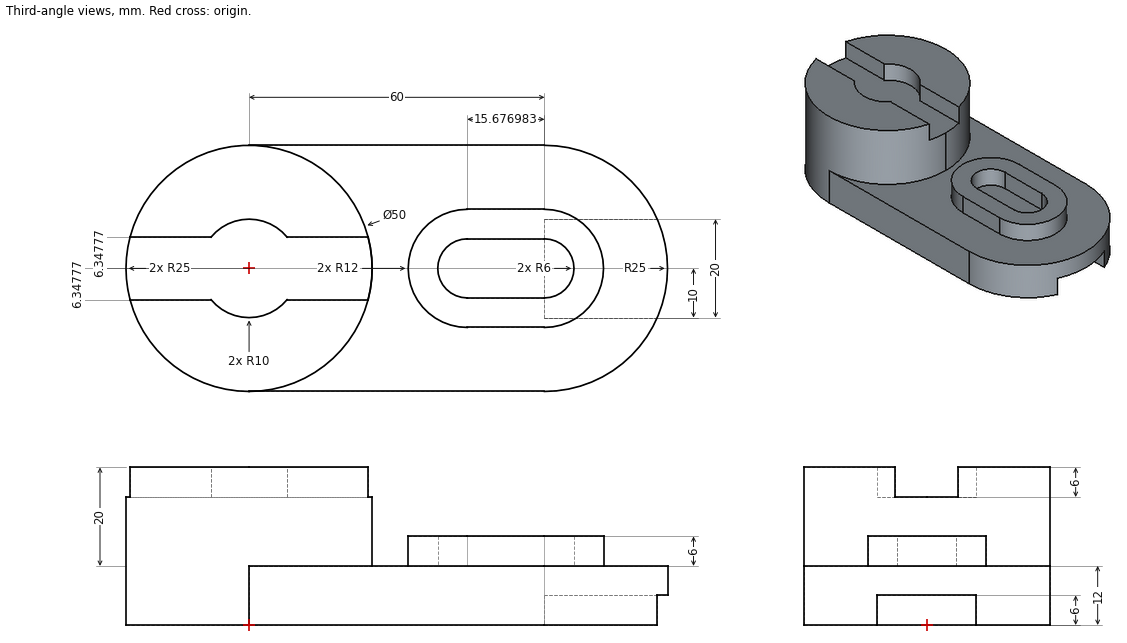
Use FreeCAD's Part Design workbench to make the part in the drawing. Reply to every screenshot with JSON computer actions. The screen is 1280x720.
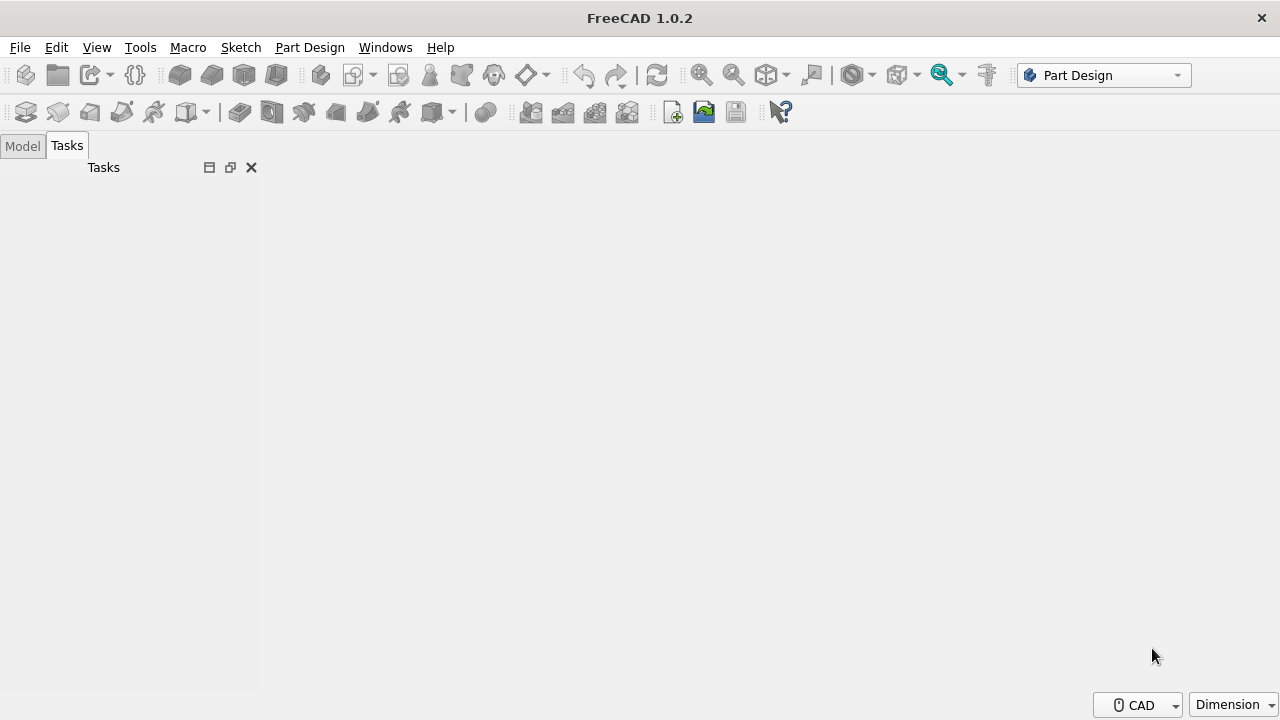
{"action": "key", "text": "ctrl+n"}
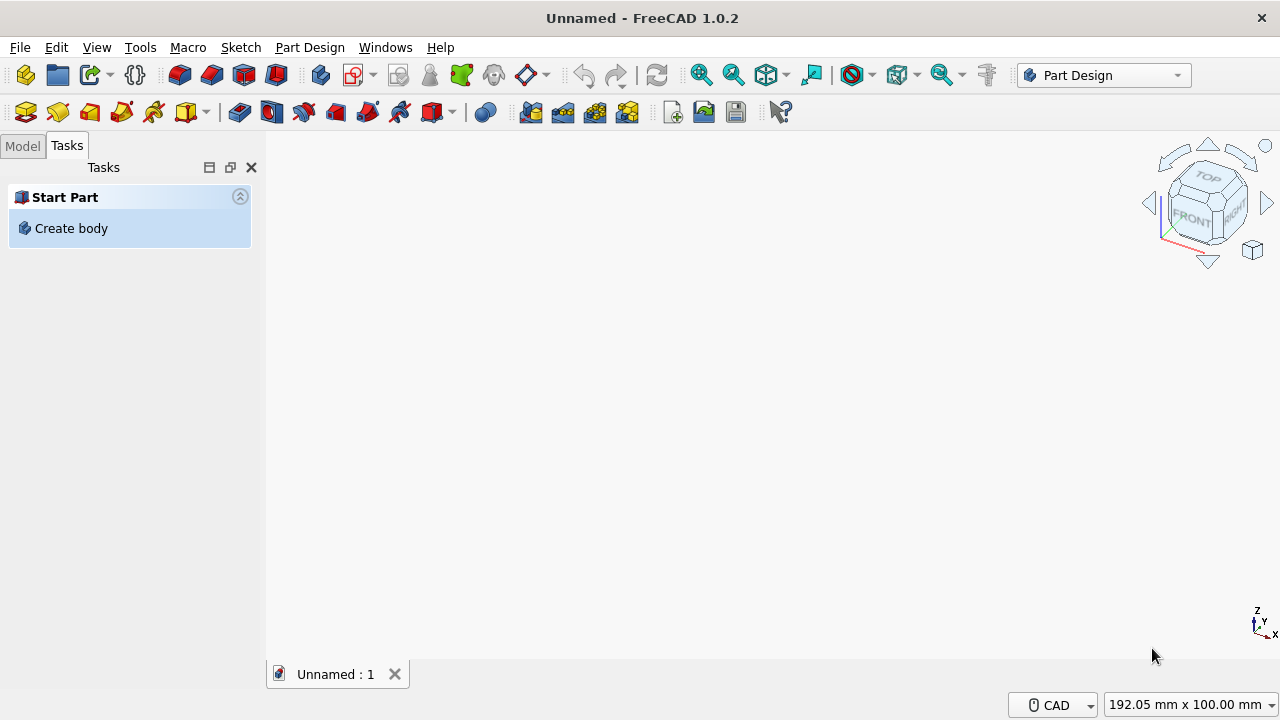
{"action": "left_click", "coordinate": [354, 76]}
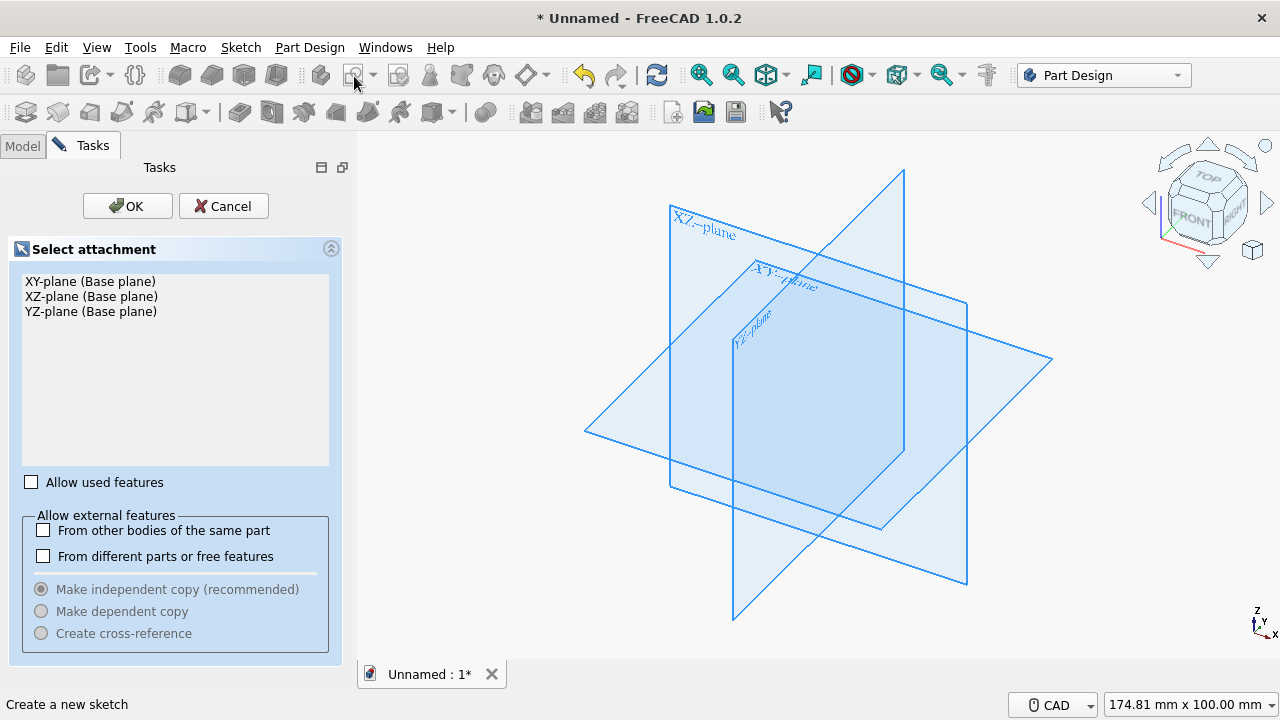
{"action": "left_click", "coordinate": [82, 282]}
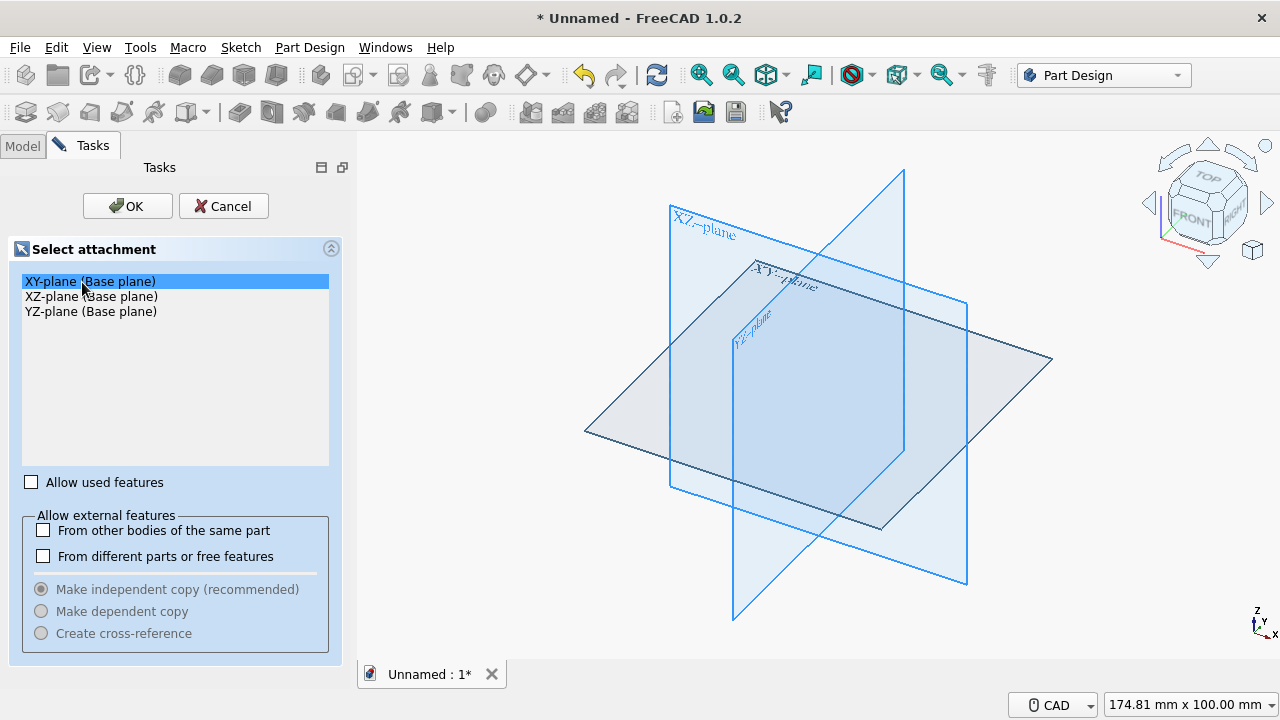
{"action": "left_click", "coordinate": [128, 206]}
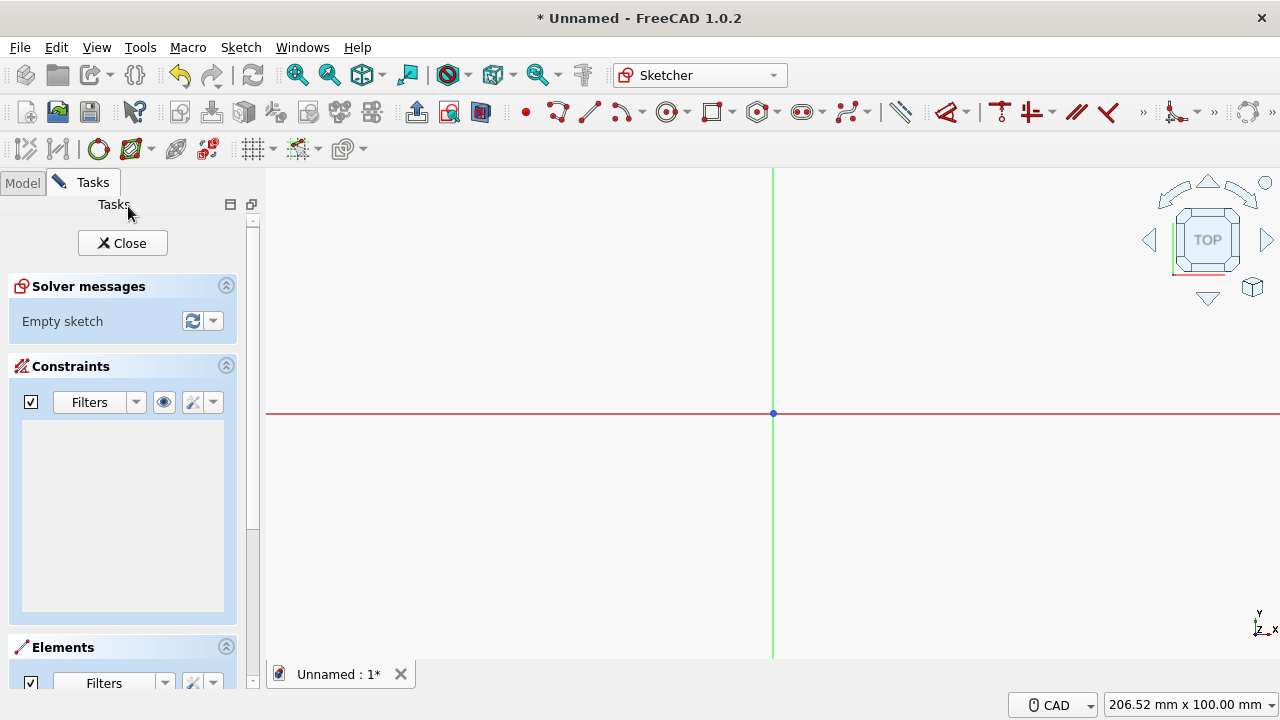
{"action": "scroll", "coordinate": [294, 413], "scroll_direction": "down", "scroll_amount": 1}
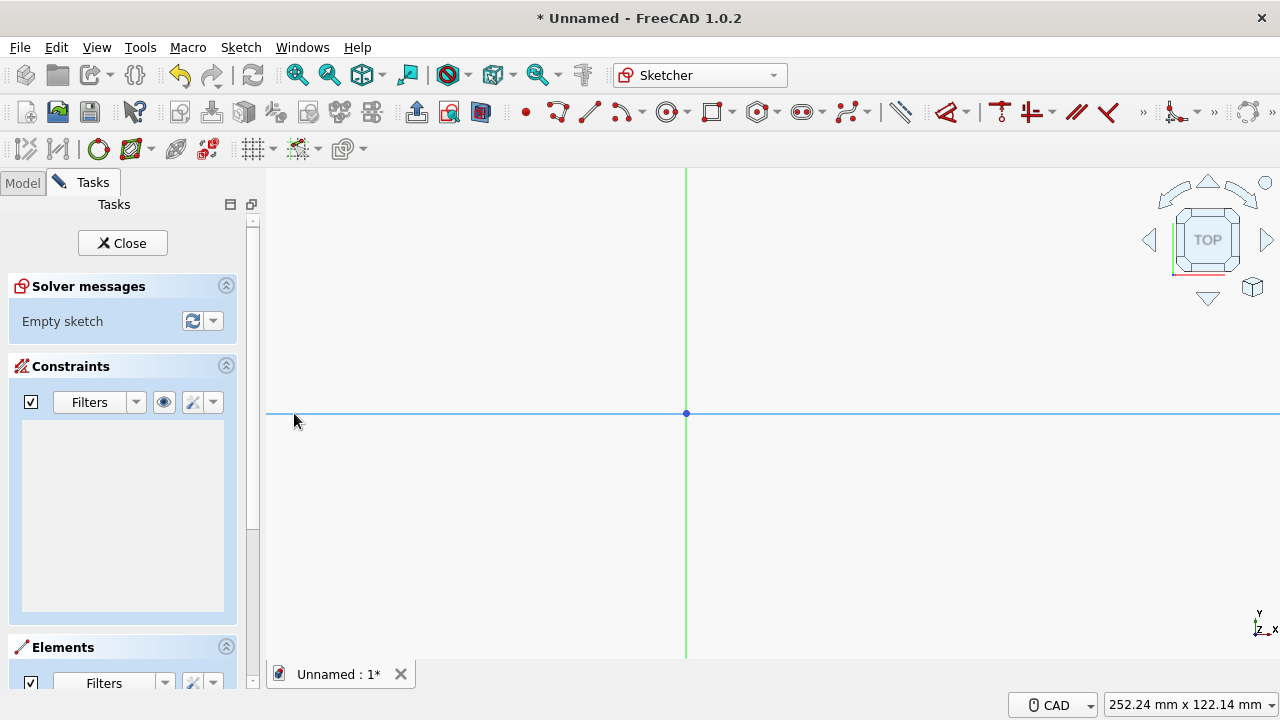
{"action": "left_click", "coordinate": [802, 112]}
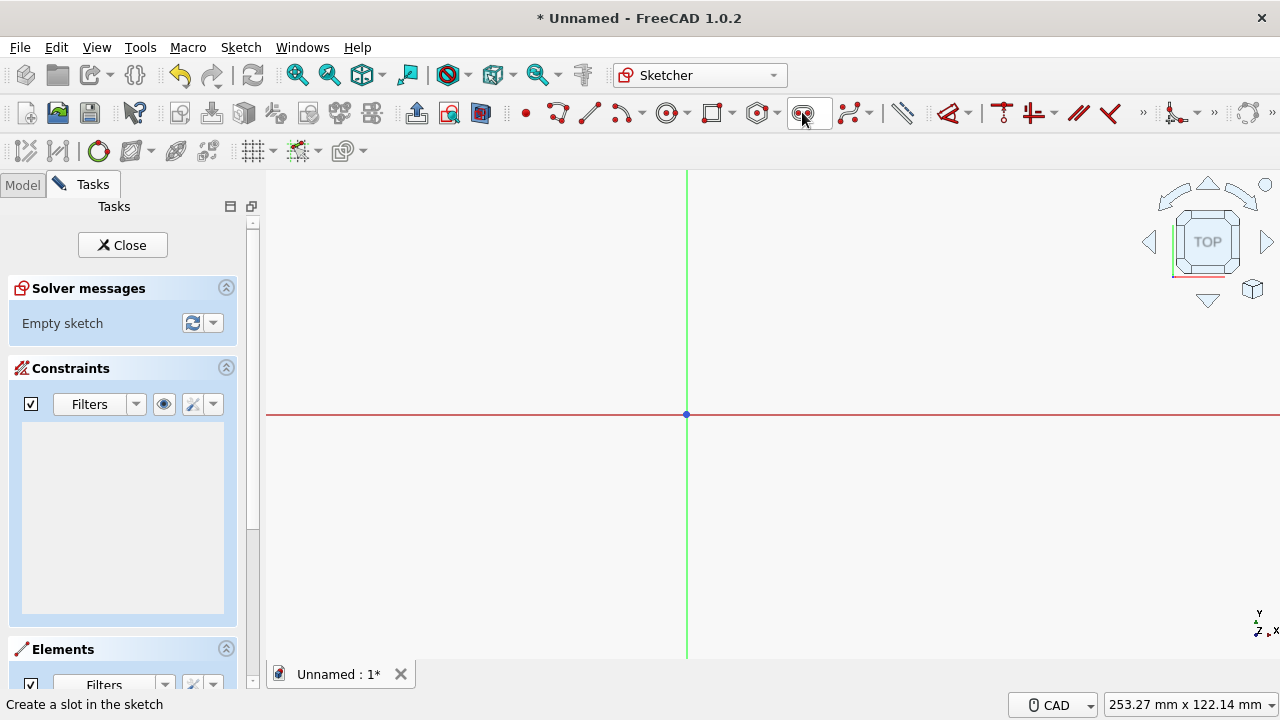
{"action": "left_click", "coordinate": [687, 414]}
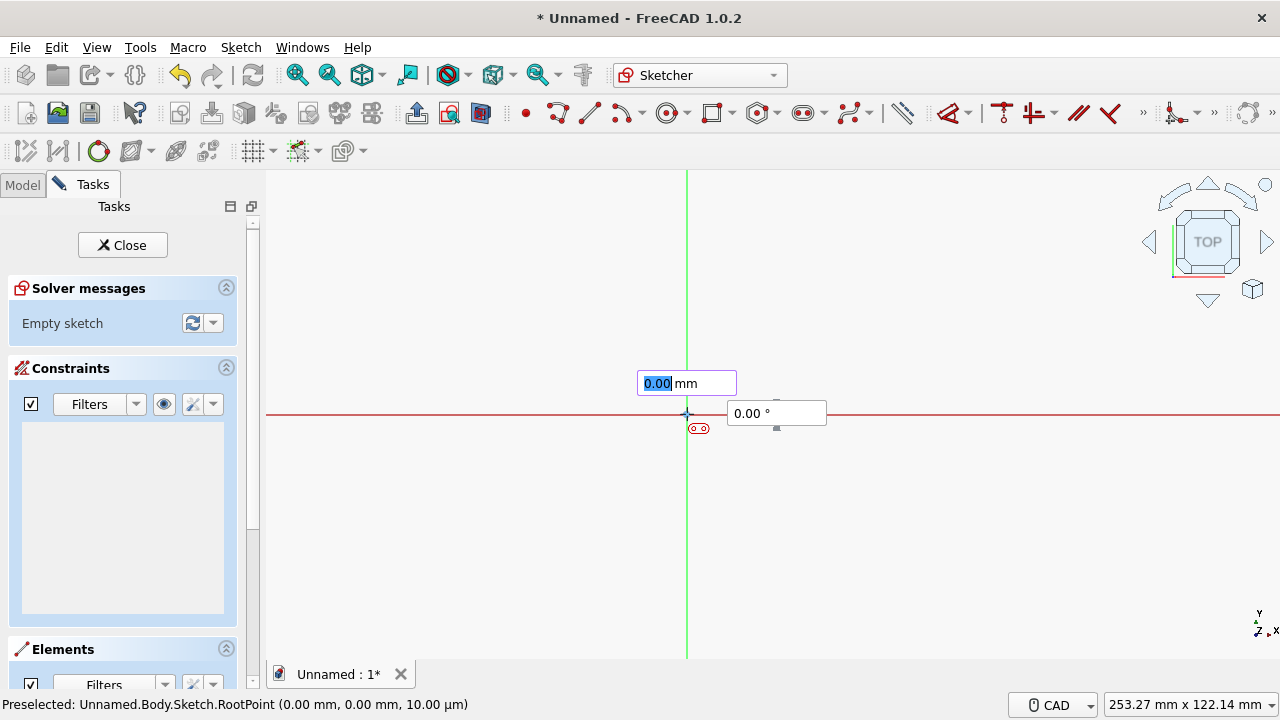
{"action": "left_click", "coordinate": [927, 406]}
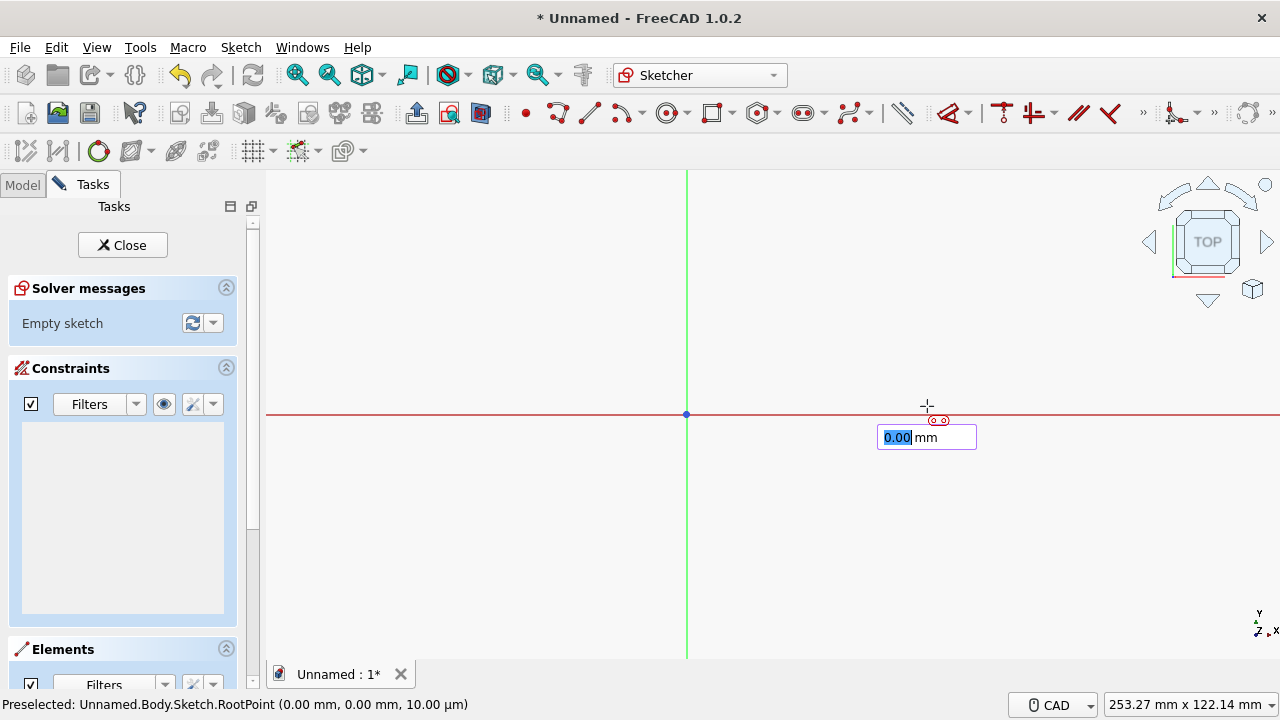
{"action": "left_click", "coordinate": [807, 314]}
{"action": "key", "text": "Escape"}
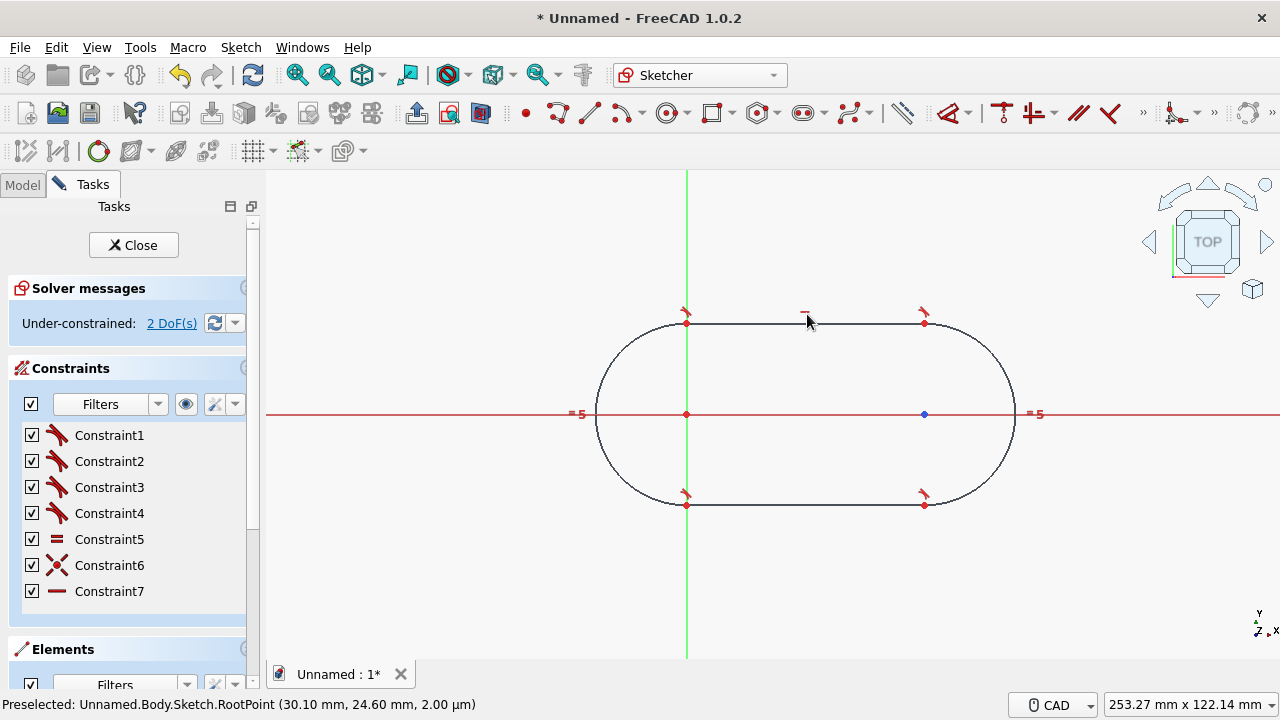
{"action": "left_click", "coordinate": [948, 114]}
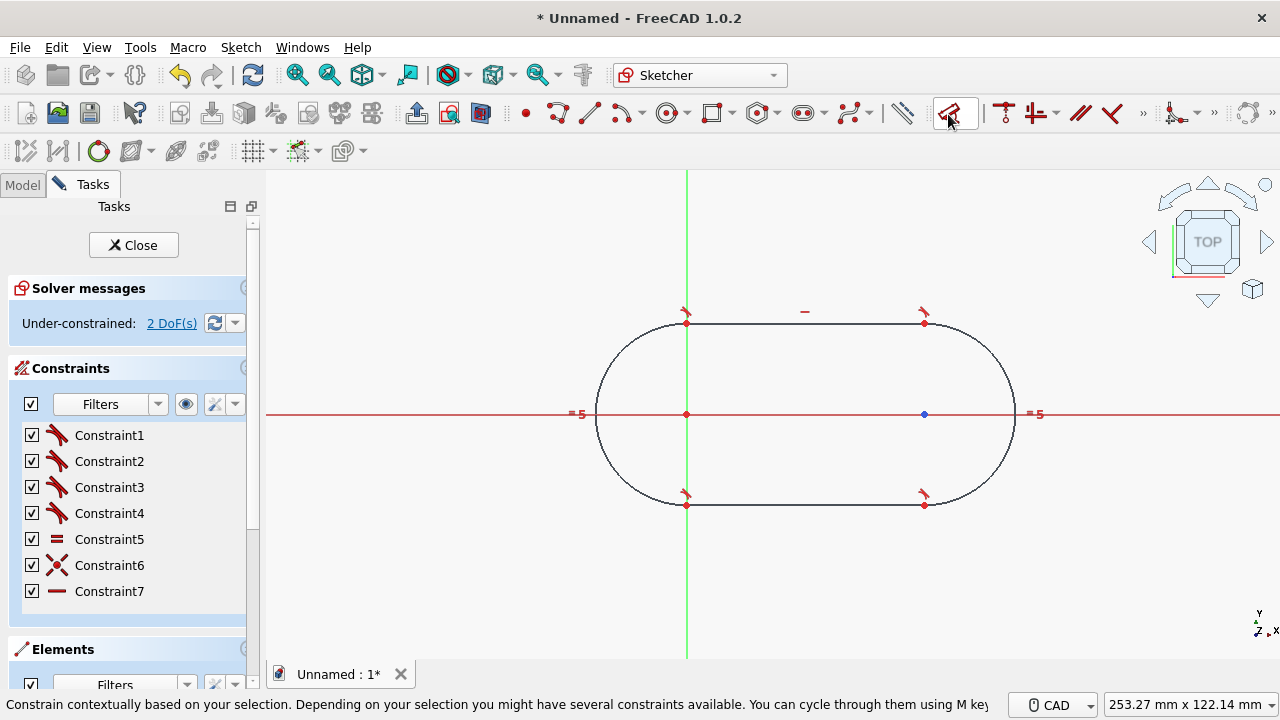
{"action": "left_click", "coordinate": [613, 361]}
{"action": "left_click", "coordinate": [587, 342]}